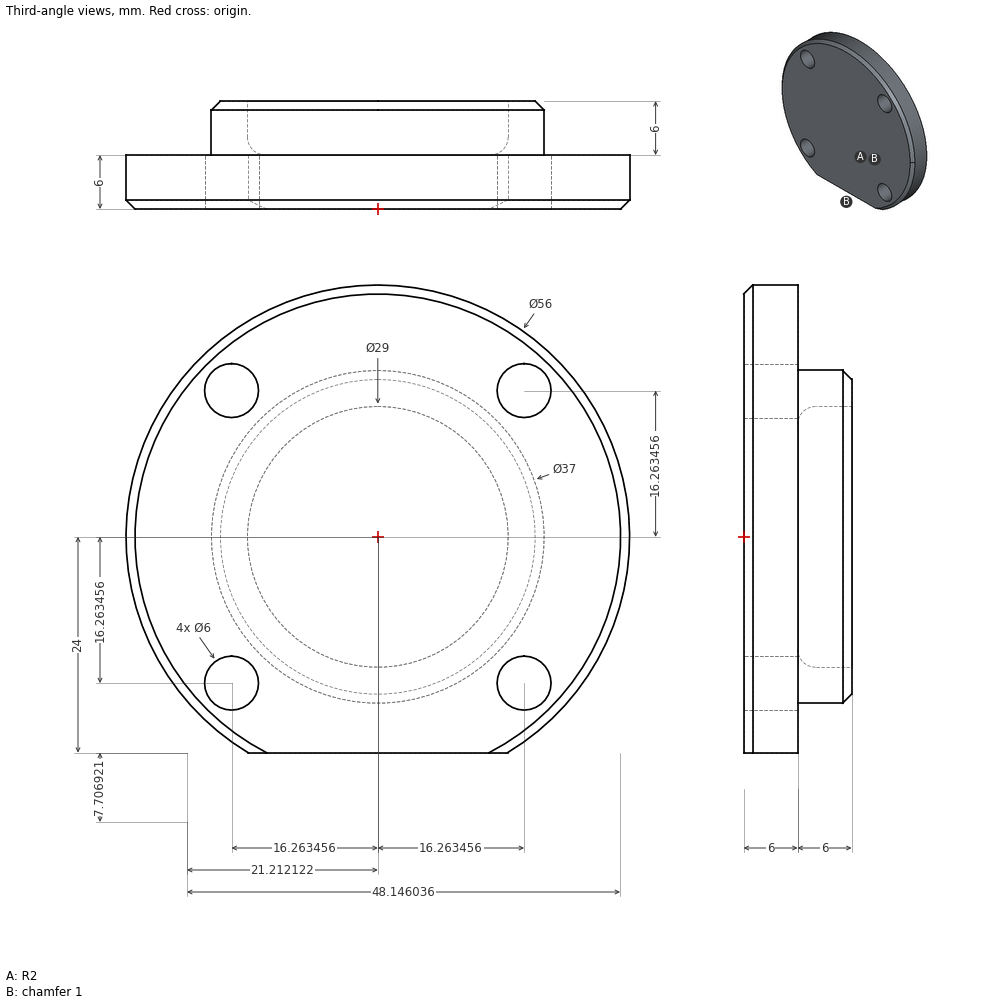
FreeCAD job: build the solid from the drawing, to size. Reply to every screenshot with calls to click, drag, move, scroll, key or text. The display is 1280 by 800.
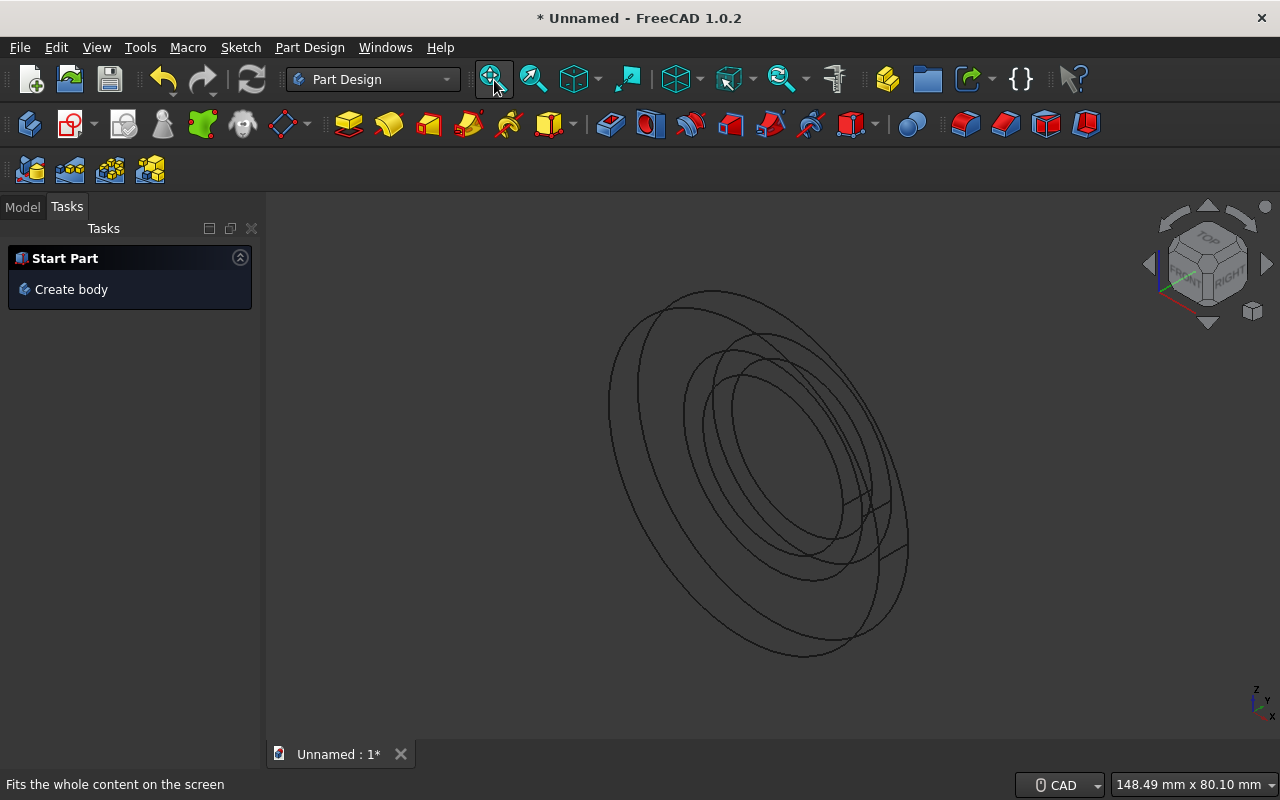
click(703, 424)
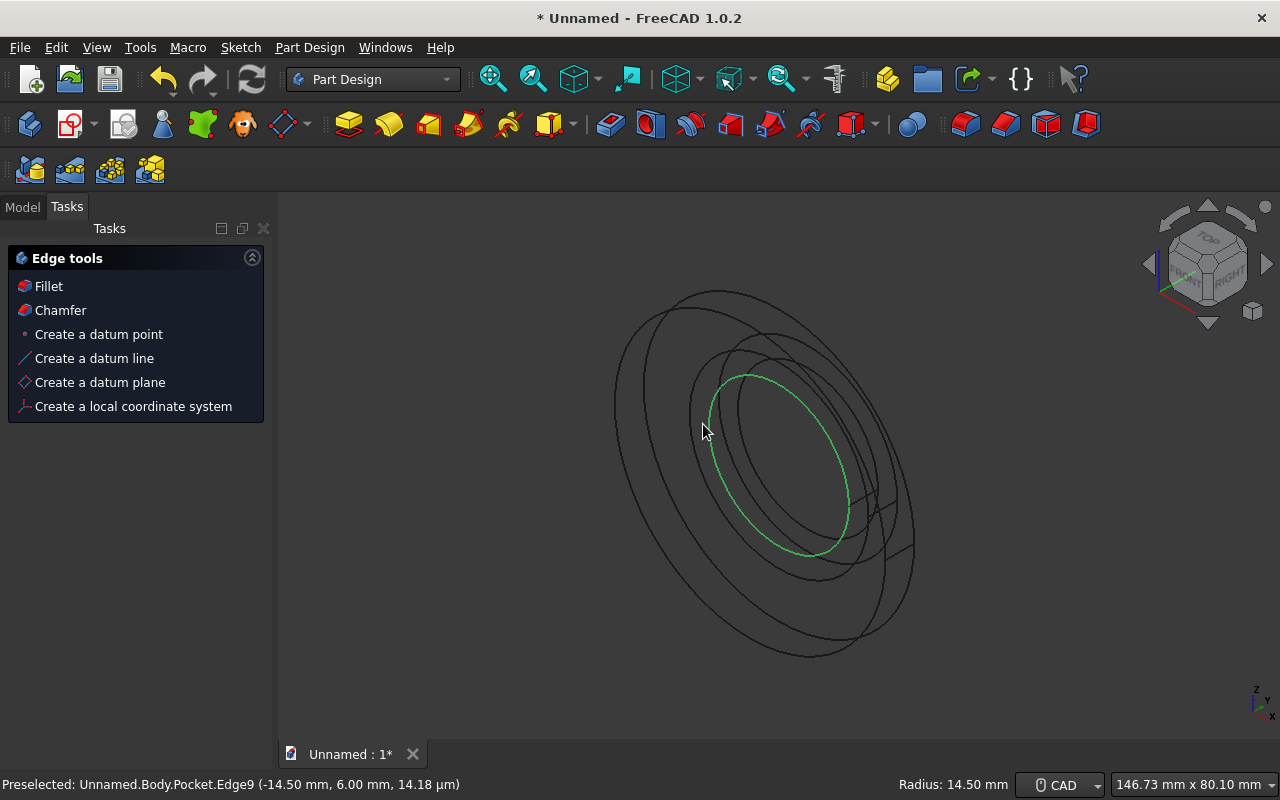
key(v)
key(1)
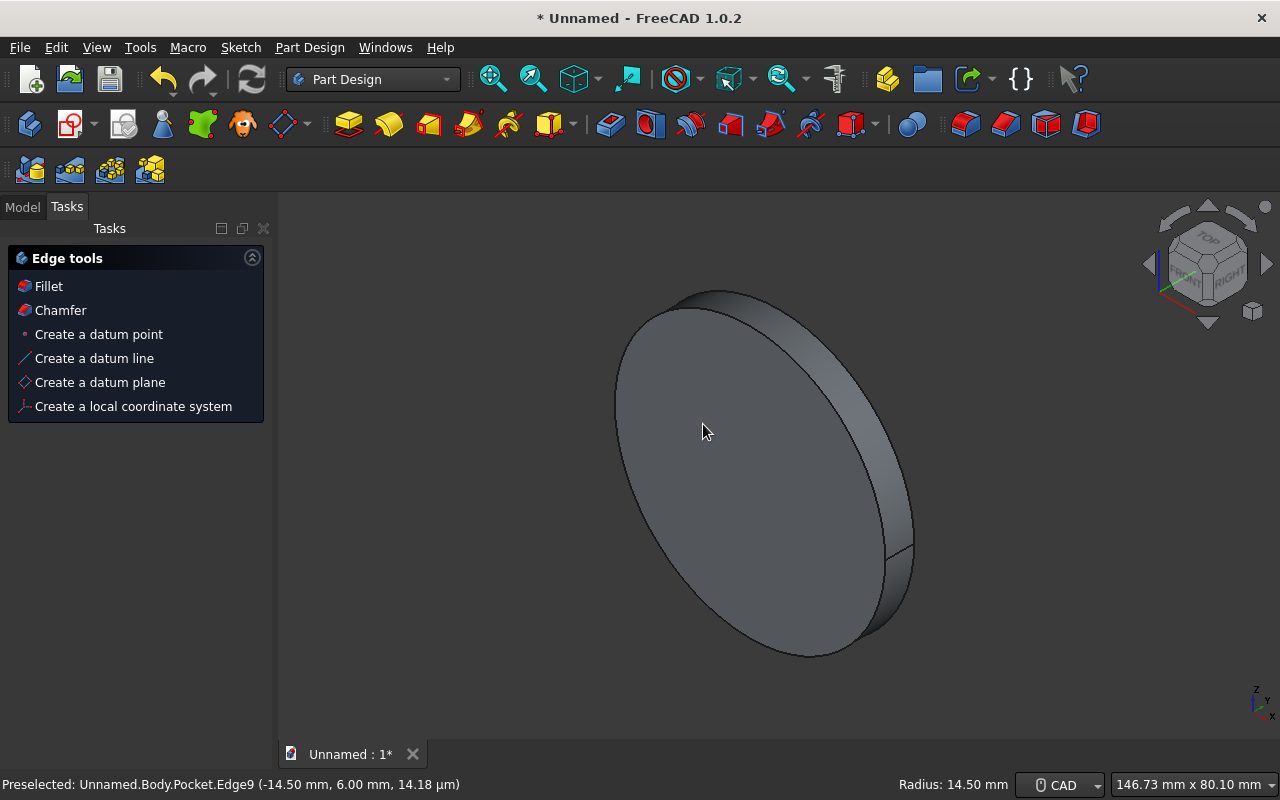
click(966, 124)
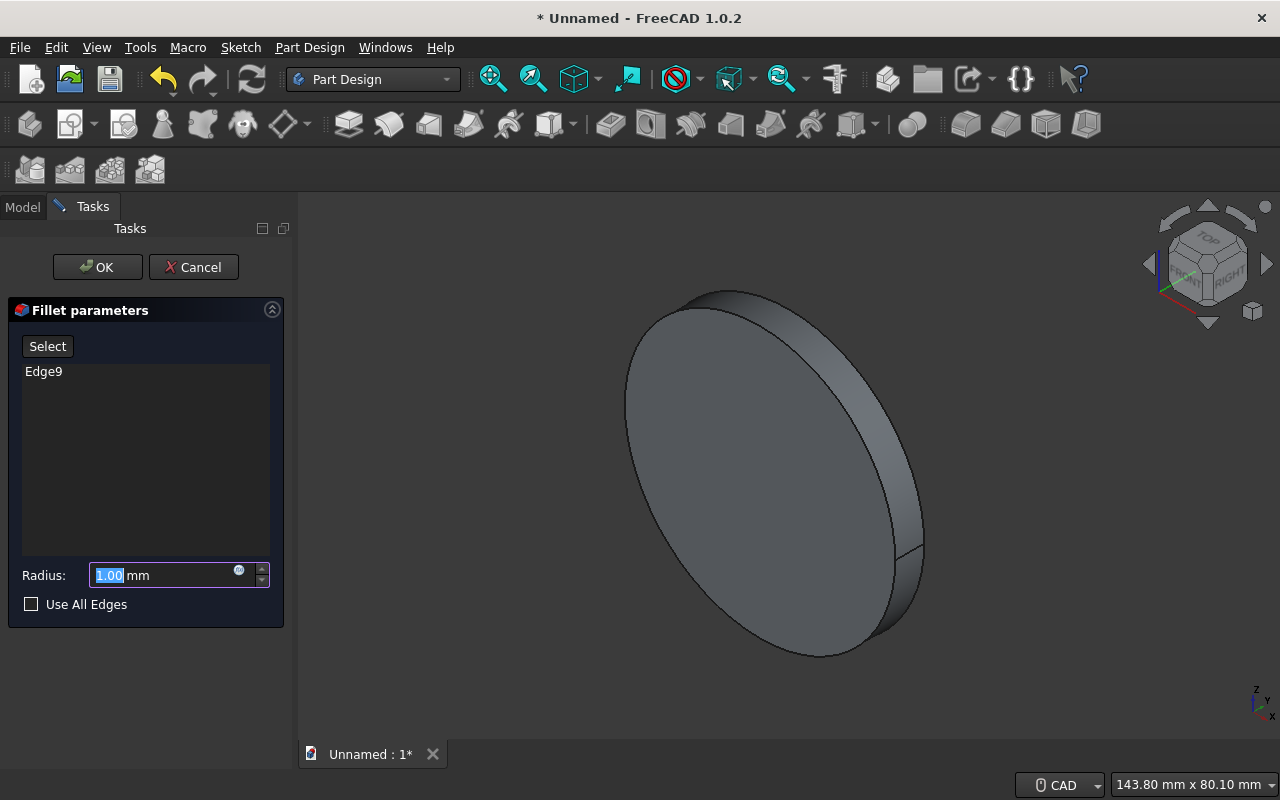
text(2)
key(Tab)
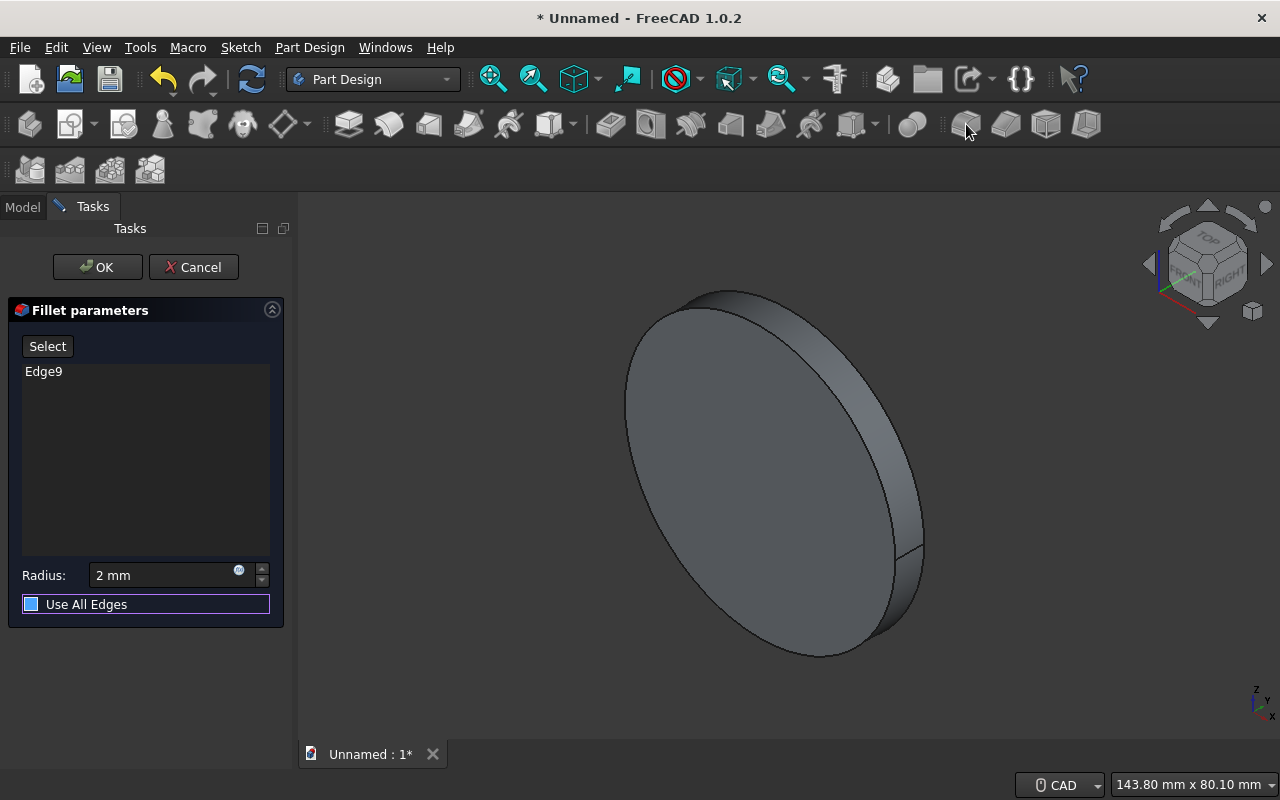
click(98, 267)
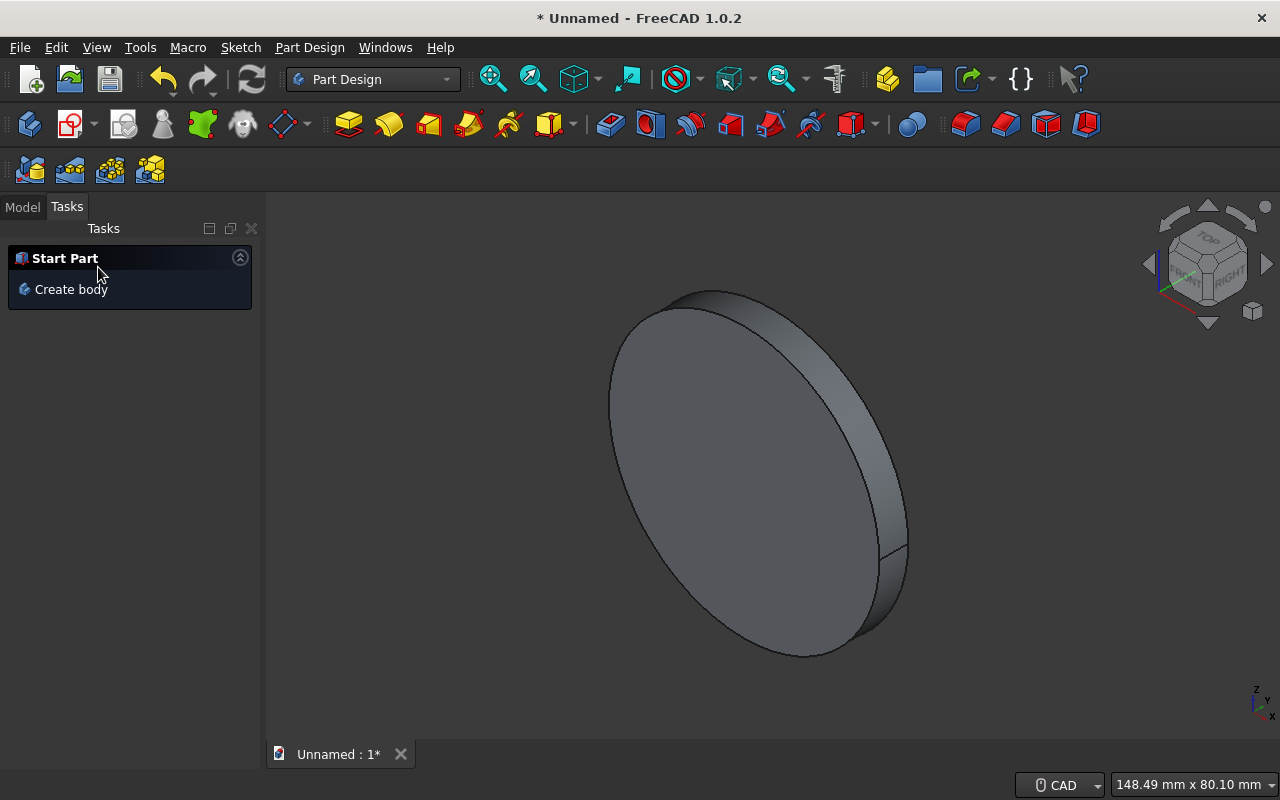
click(702, 309)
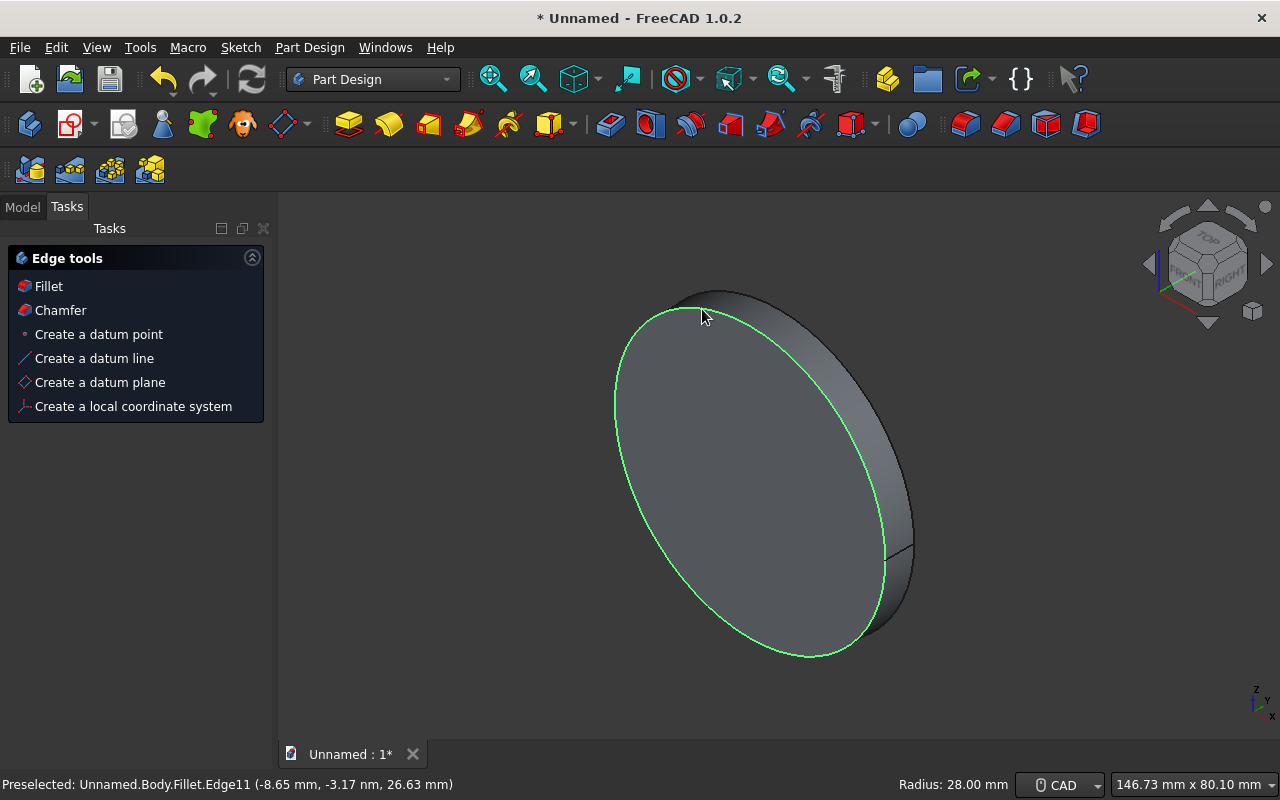
key(2)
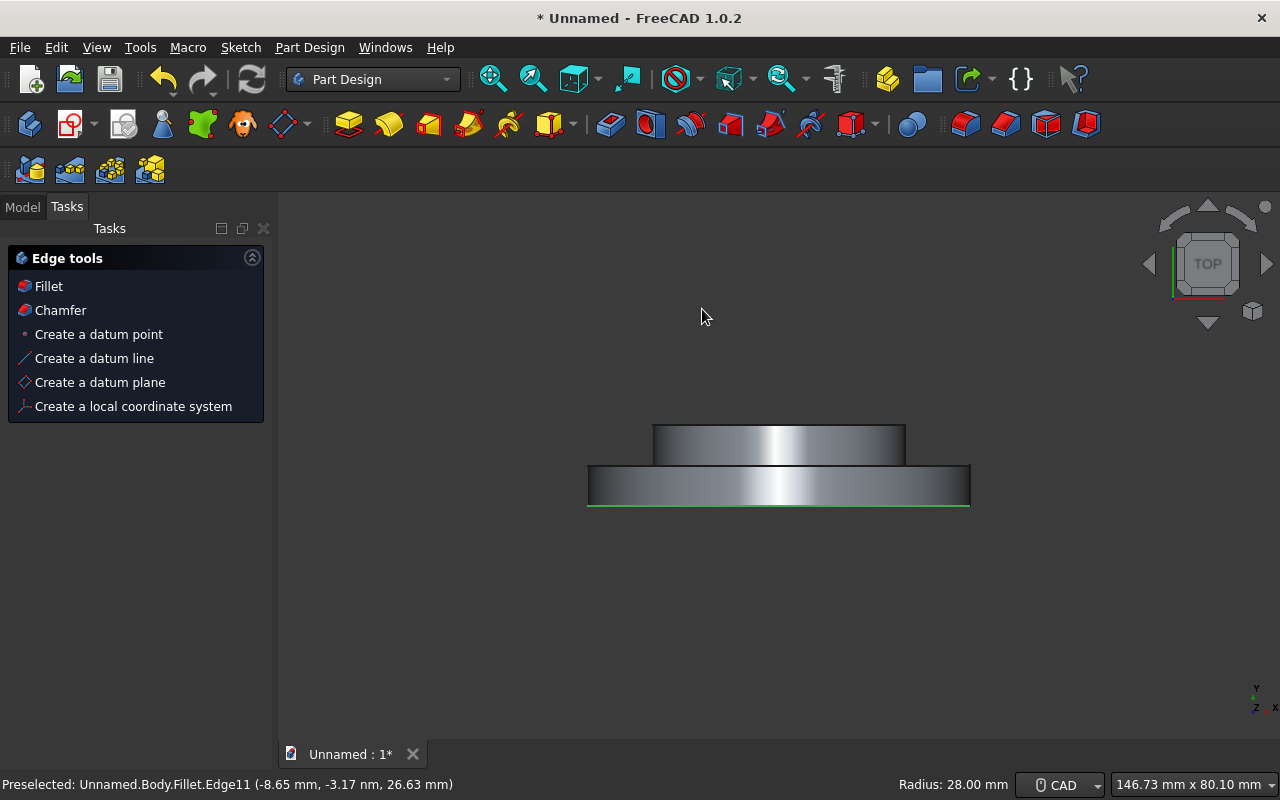
click(494, 80)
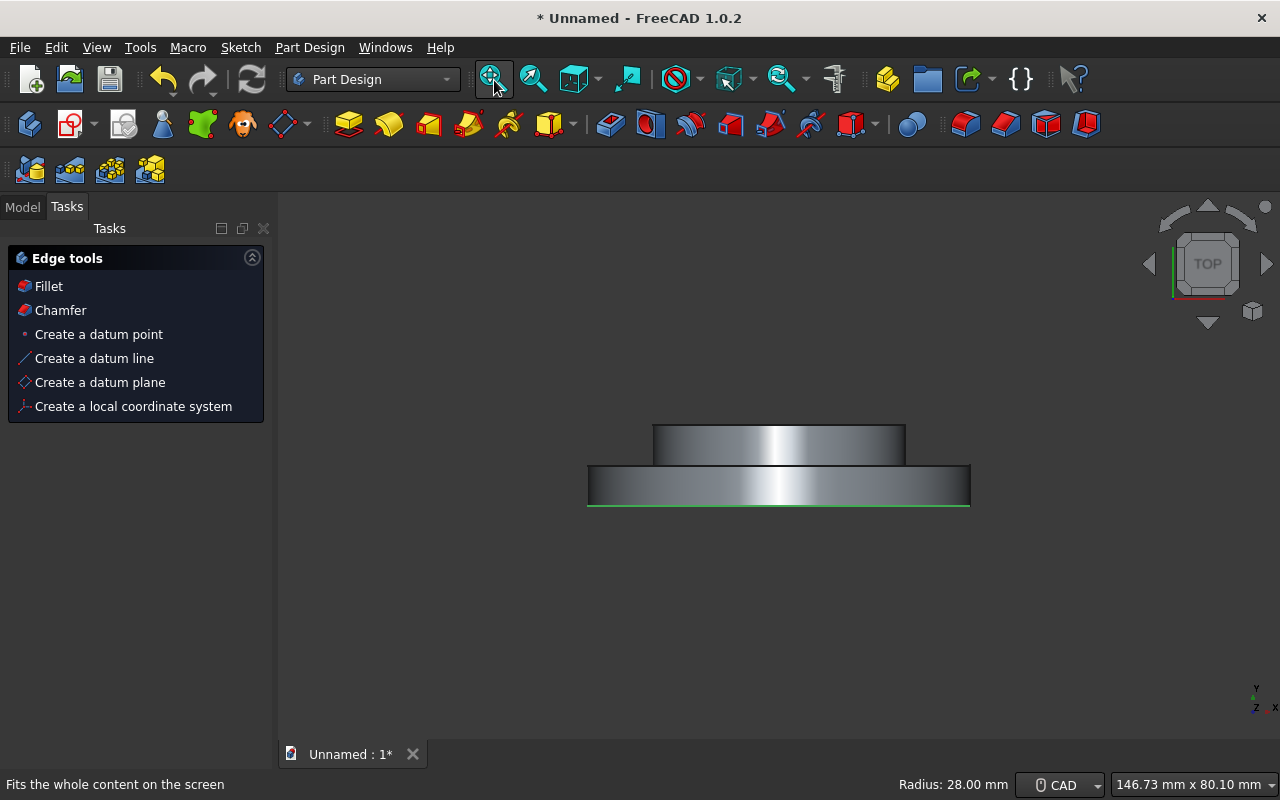
click(677, 424, ctrl)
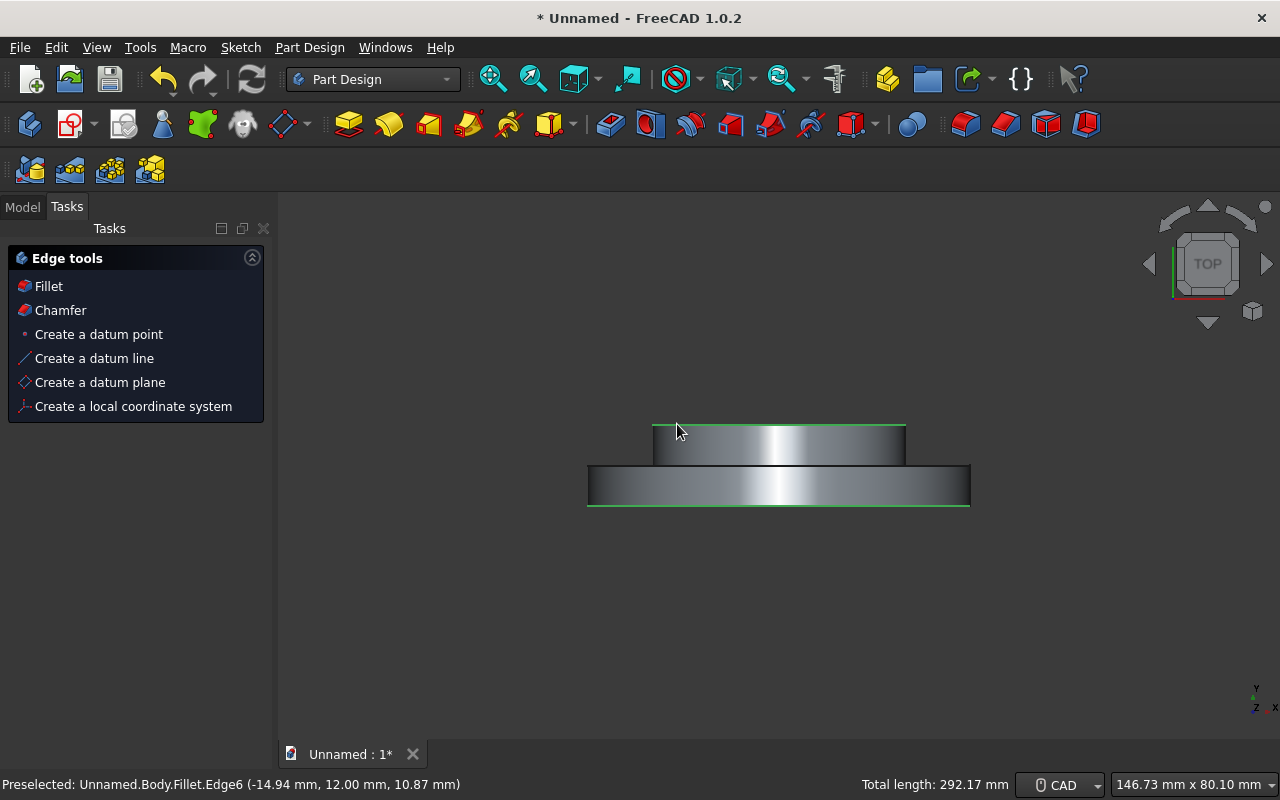
click(1006, 124)